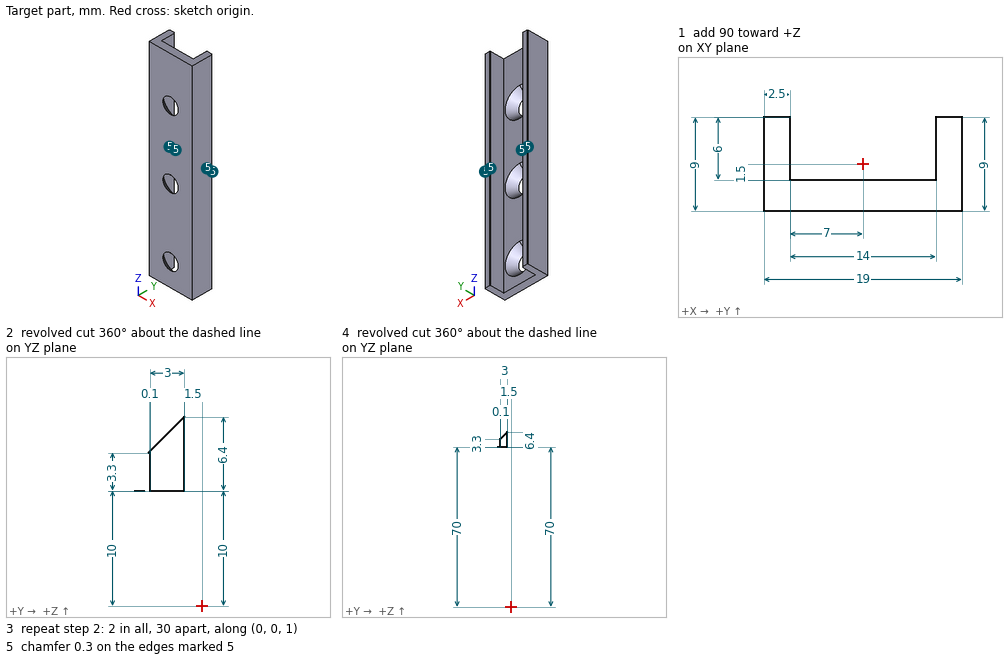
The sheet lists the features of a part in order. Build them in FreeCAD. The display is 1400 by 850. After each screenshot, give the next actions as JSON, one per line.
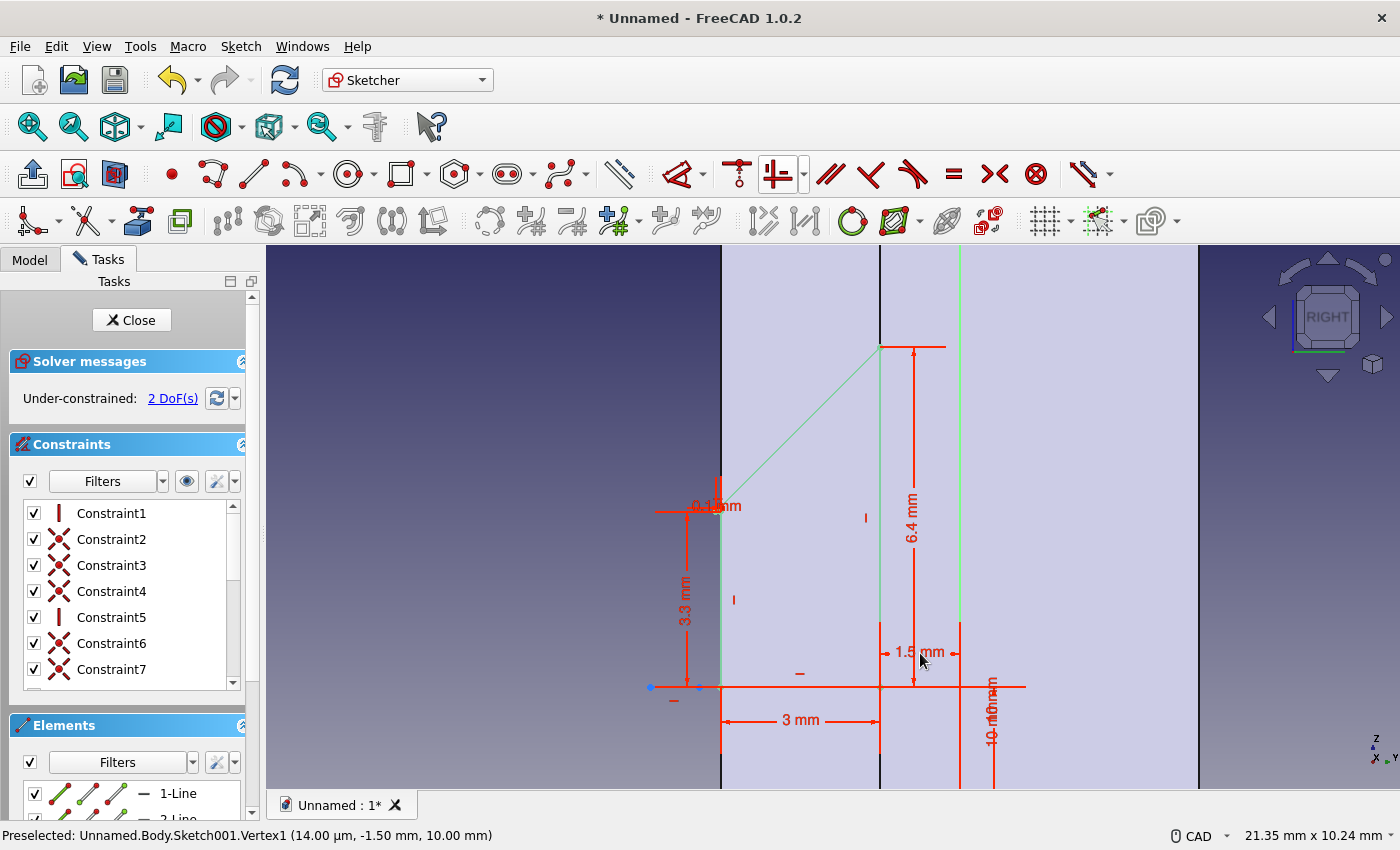
{"action": "left_click", "coordinate": [132, 320]}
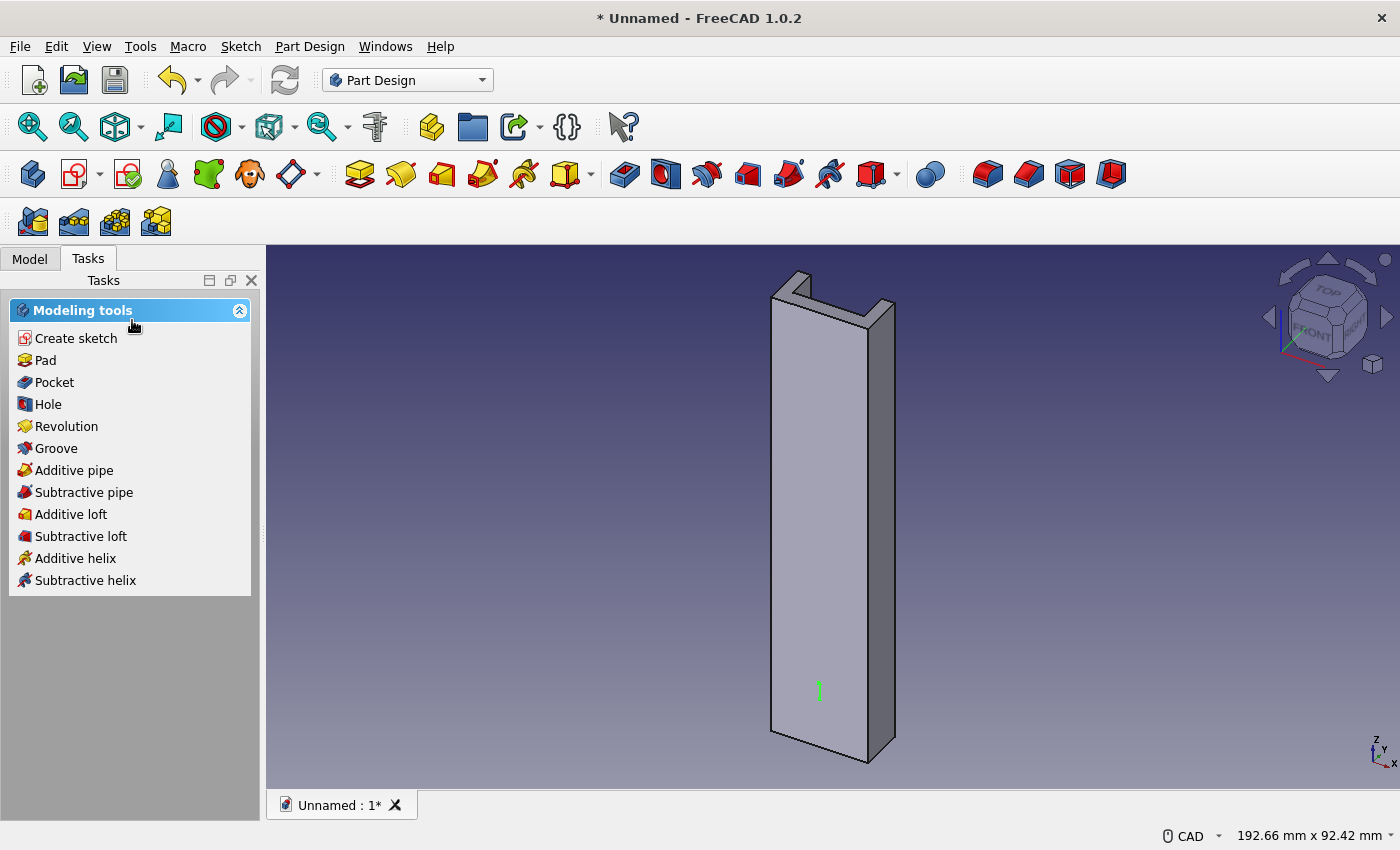
{"action": "left_click", "coordinate": [707, 174]}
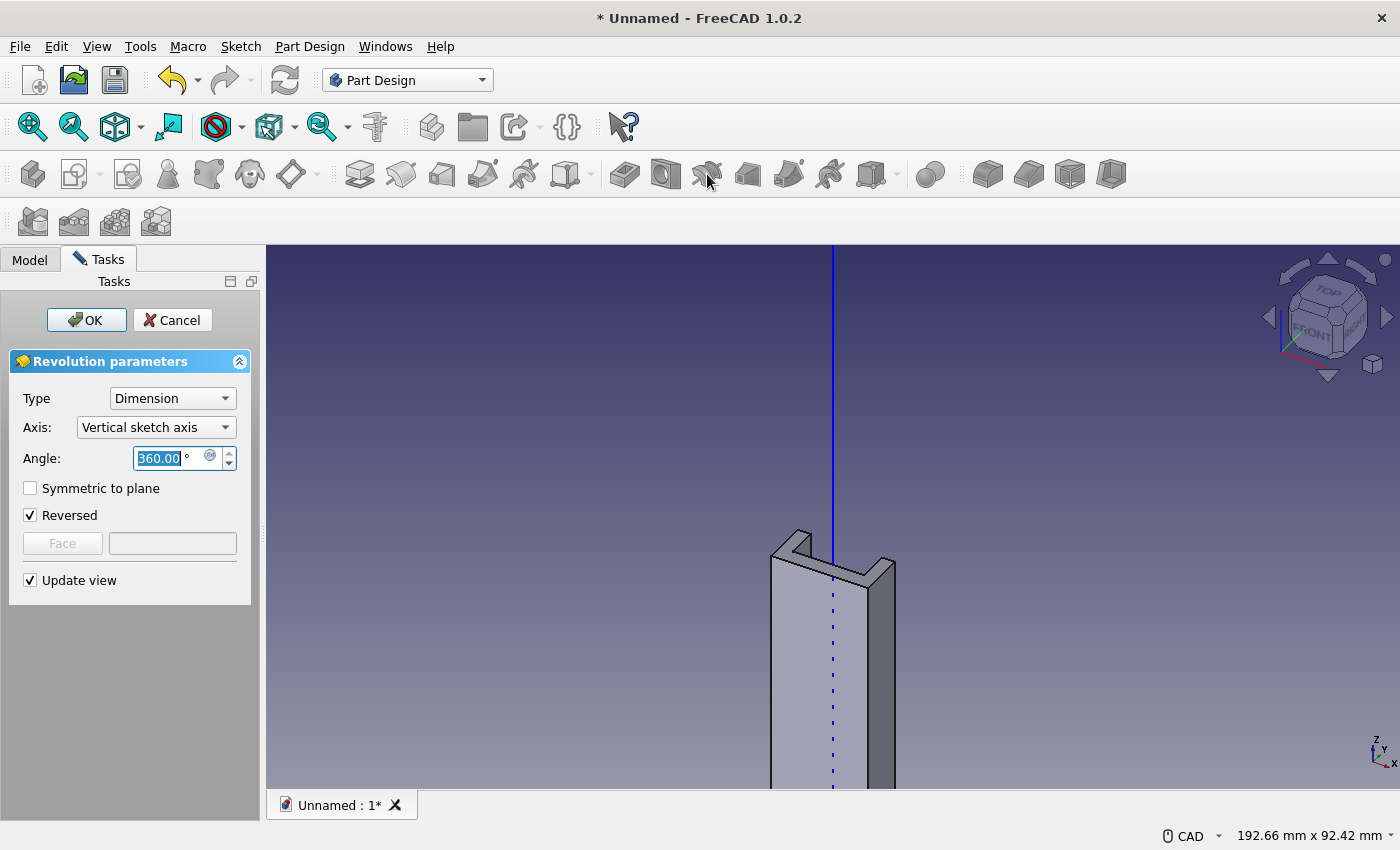
{"action": "left_click", "coordinate": [157, 428]}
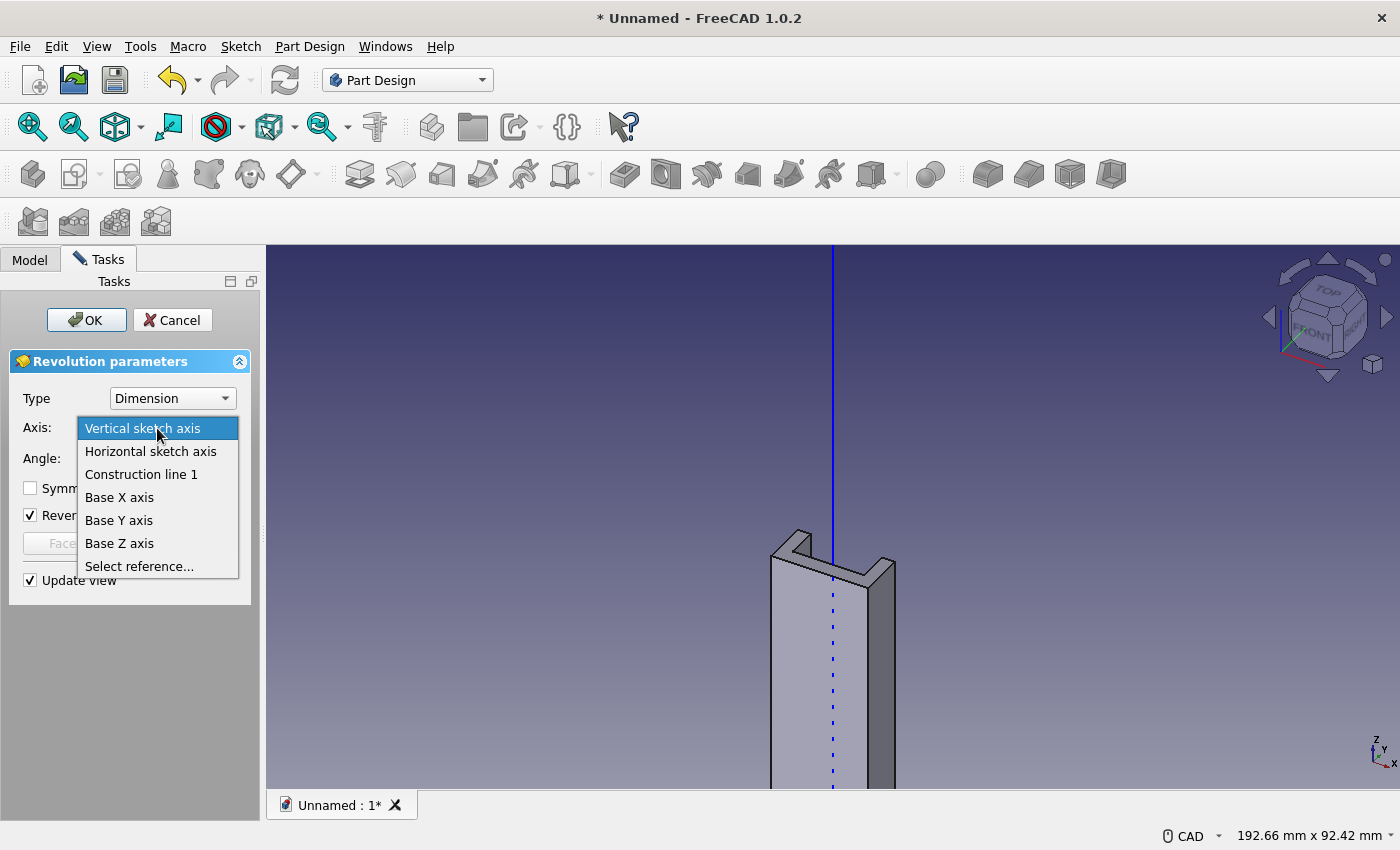
{"action": "left_click", "coordinate": [156, 474]}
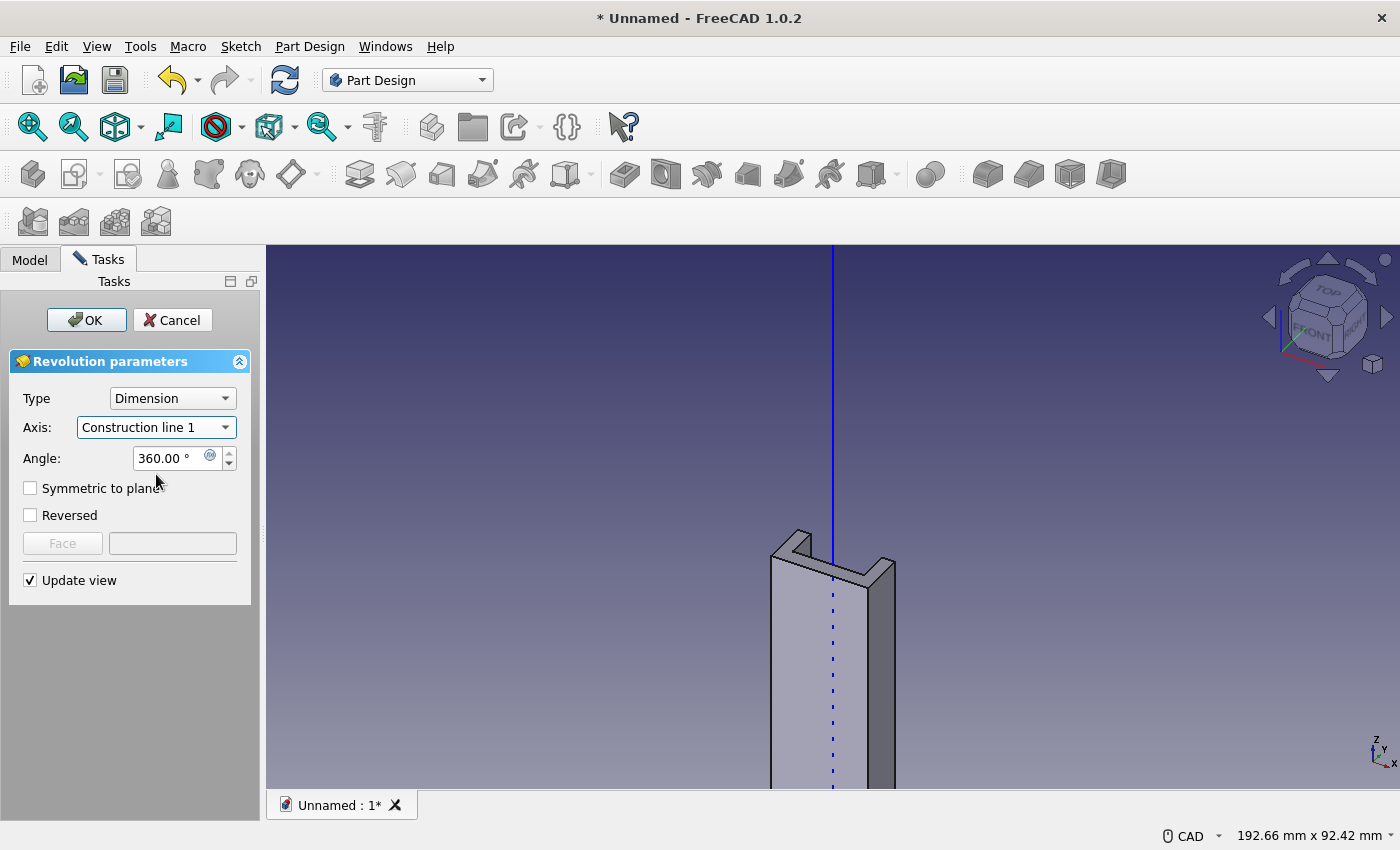
{"action": "left_click", "coordinate": [87, 320]}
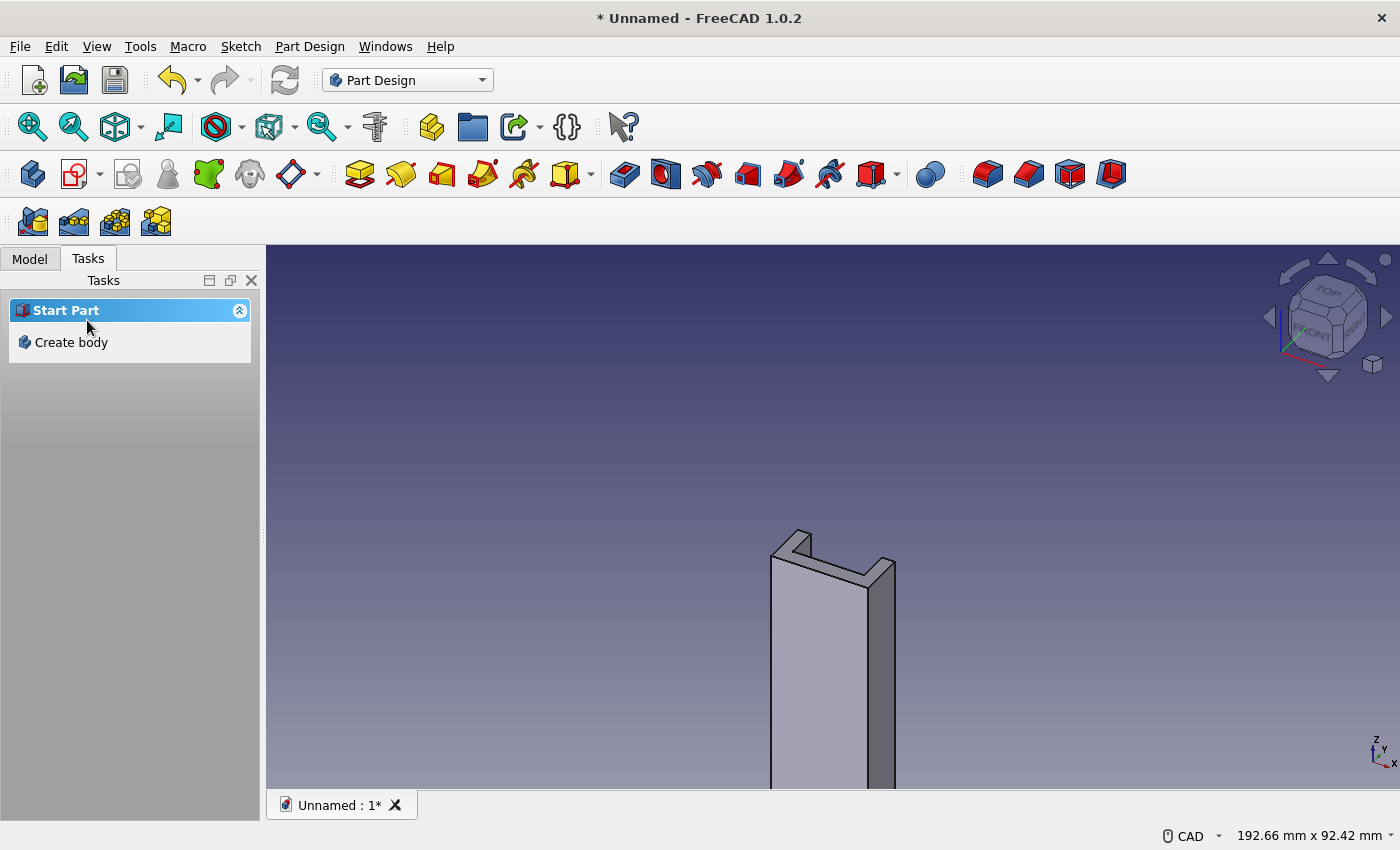
{"action": "left_click", "coordinate": [33, 128]}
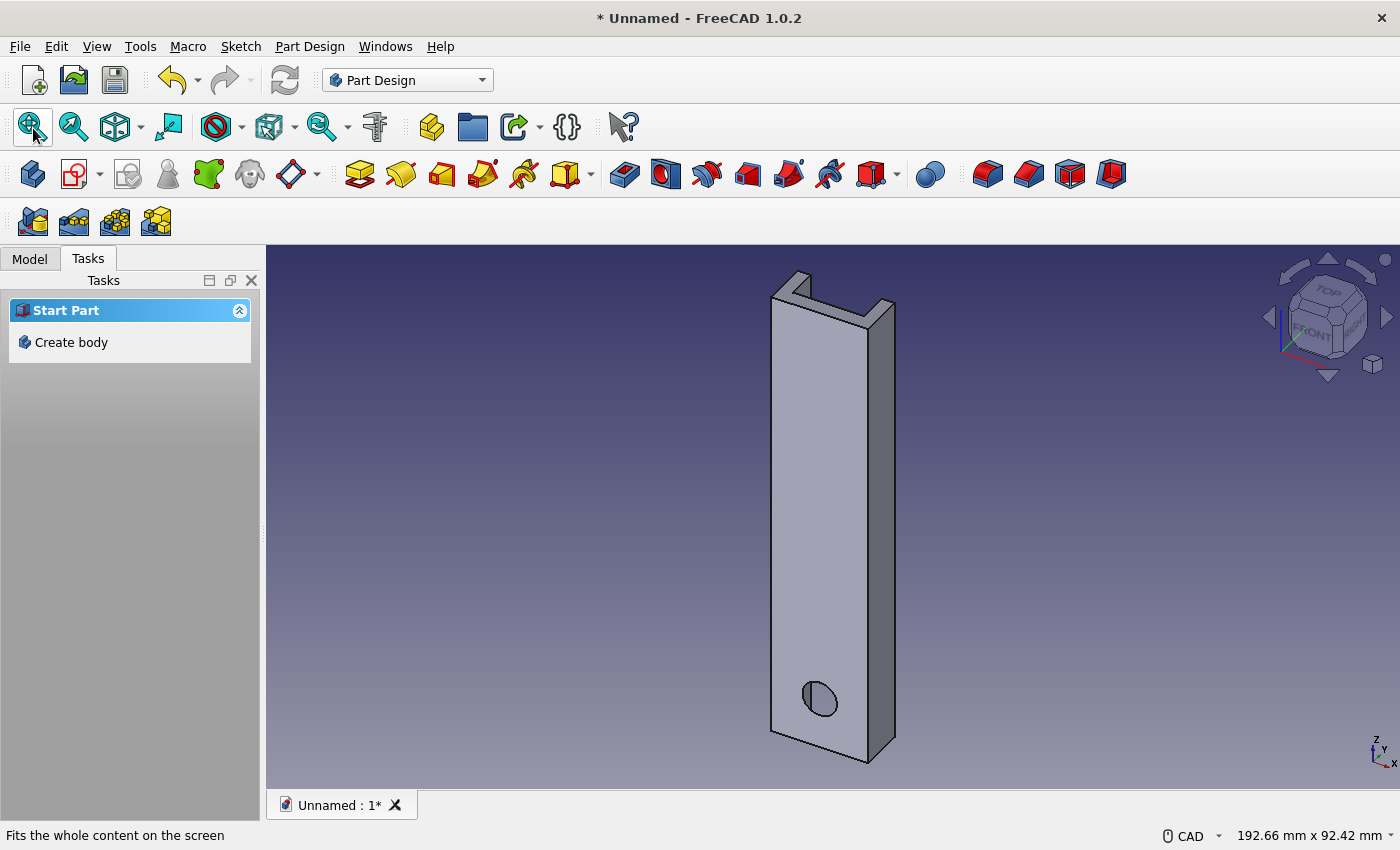
{"action": "left_click", "coordinate": [30, 258]}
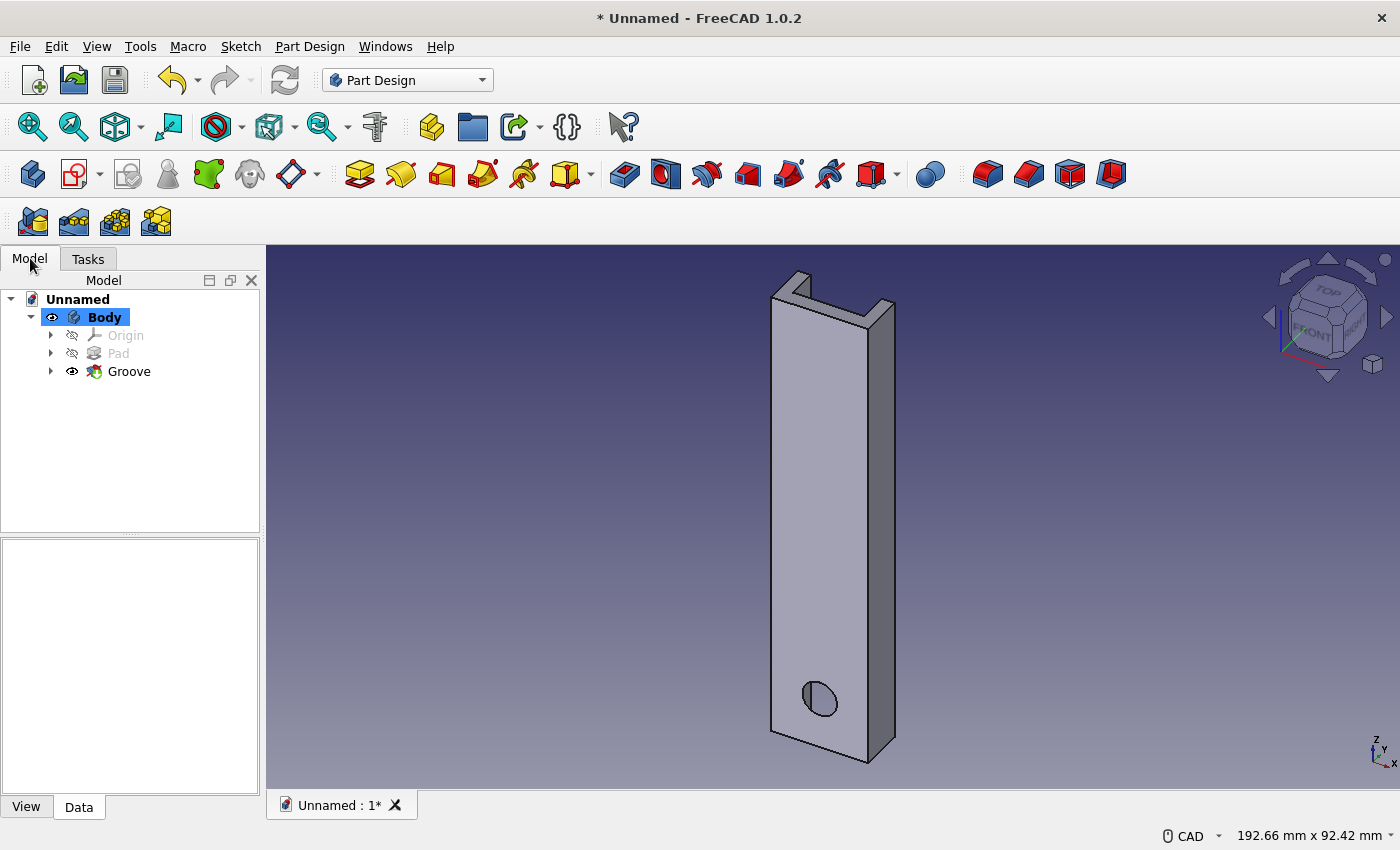
{"action": "left_click", "coordinate": [117, 371]}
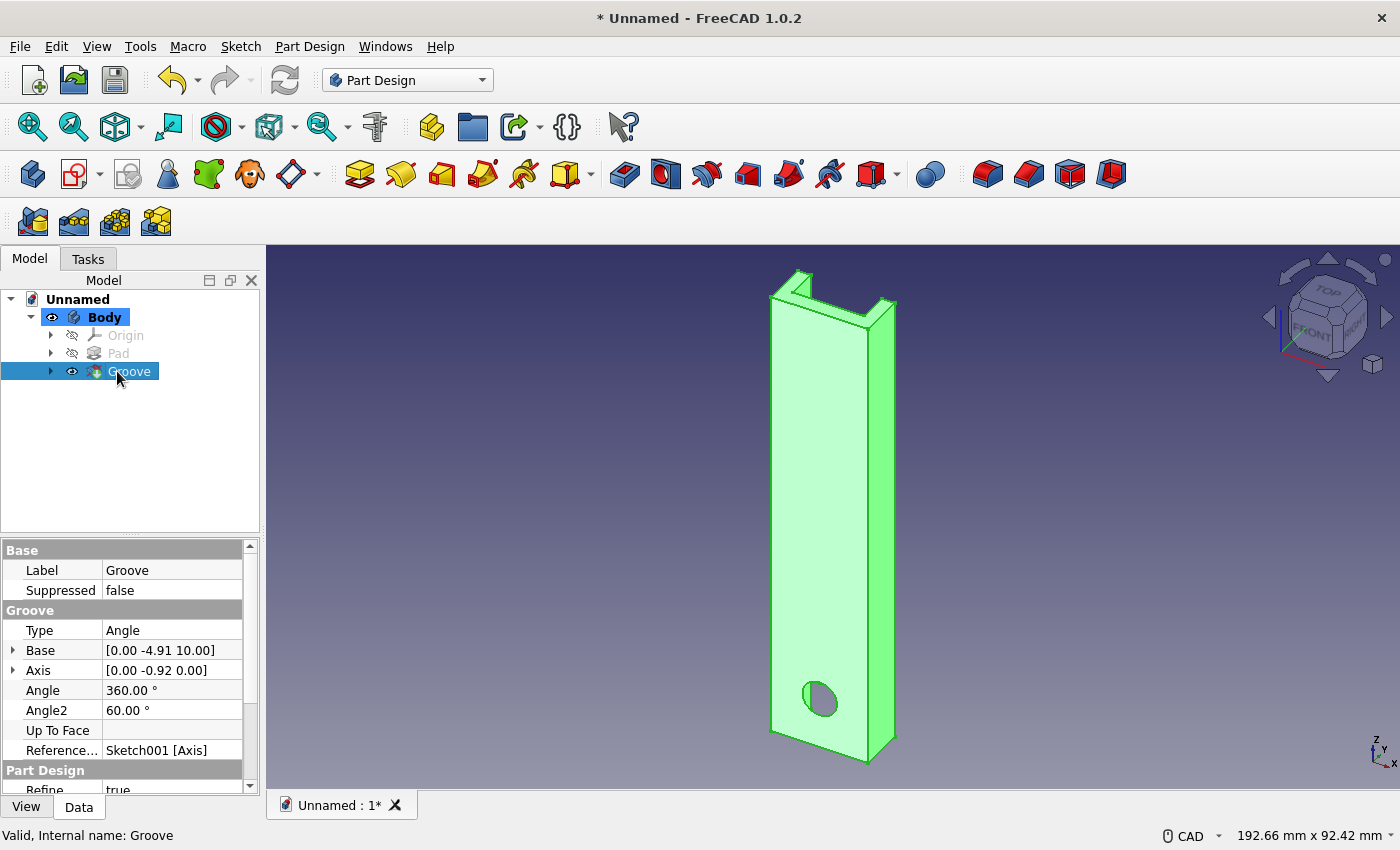
{"action": "left_click", "coordinate": [74, 222]}